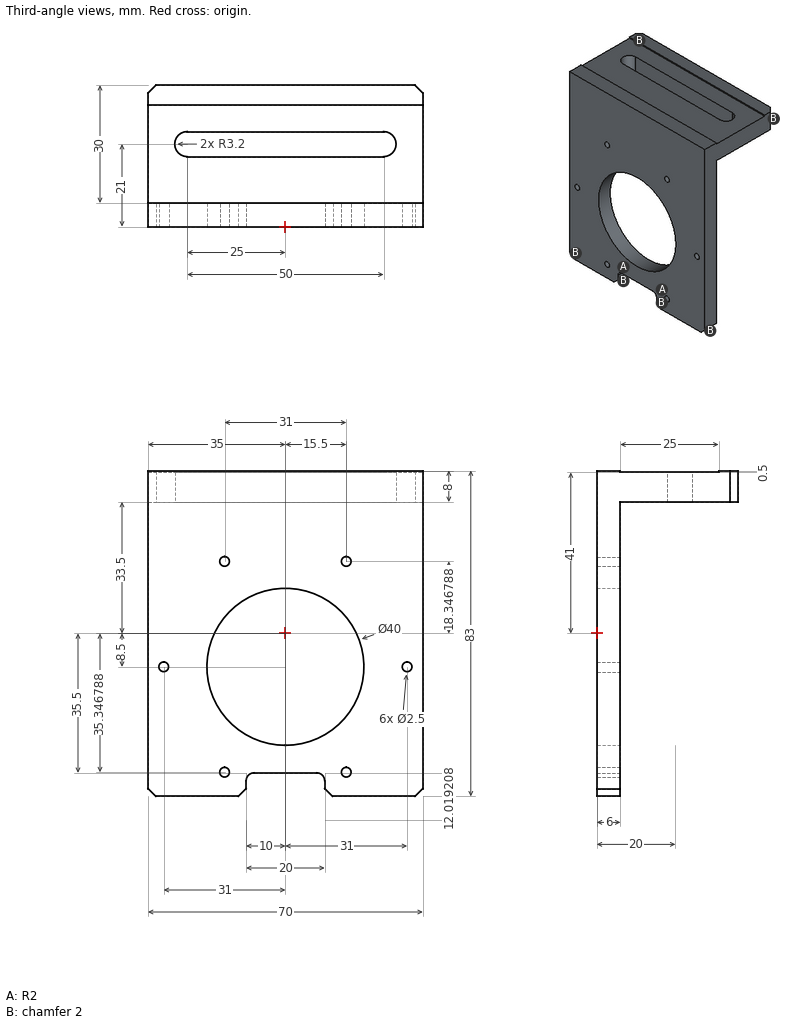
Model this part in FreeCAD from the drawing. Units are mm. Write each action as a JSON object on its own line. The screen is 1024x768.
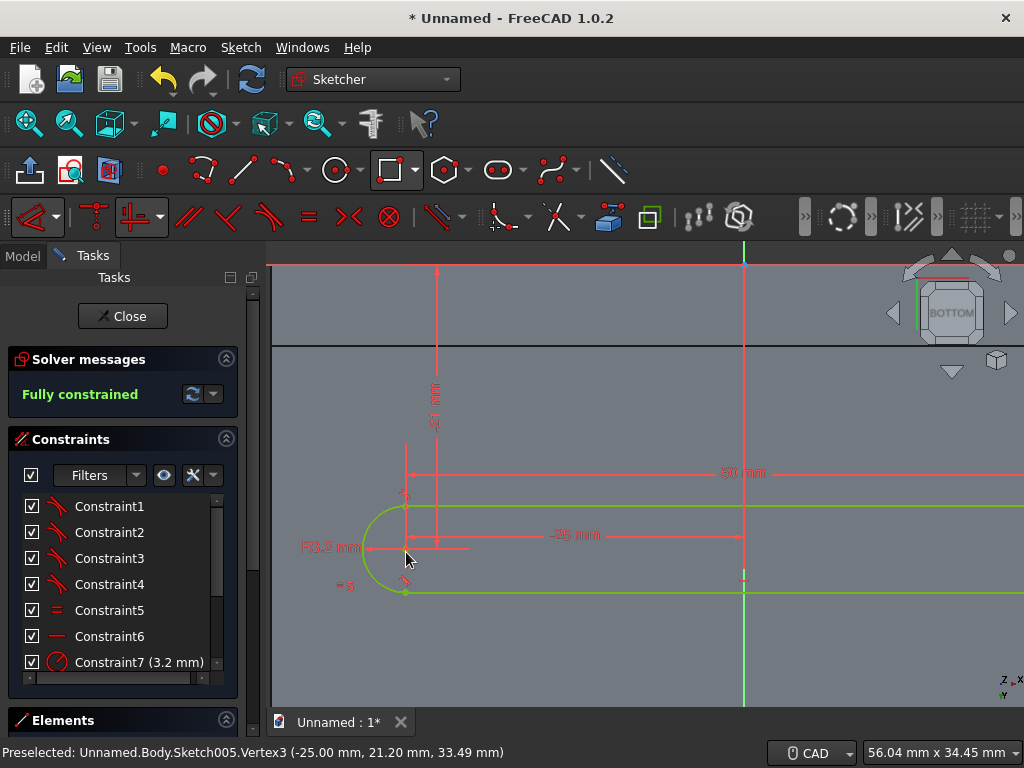
{"action": "left_click", "coordinate": [123, 316]}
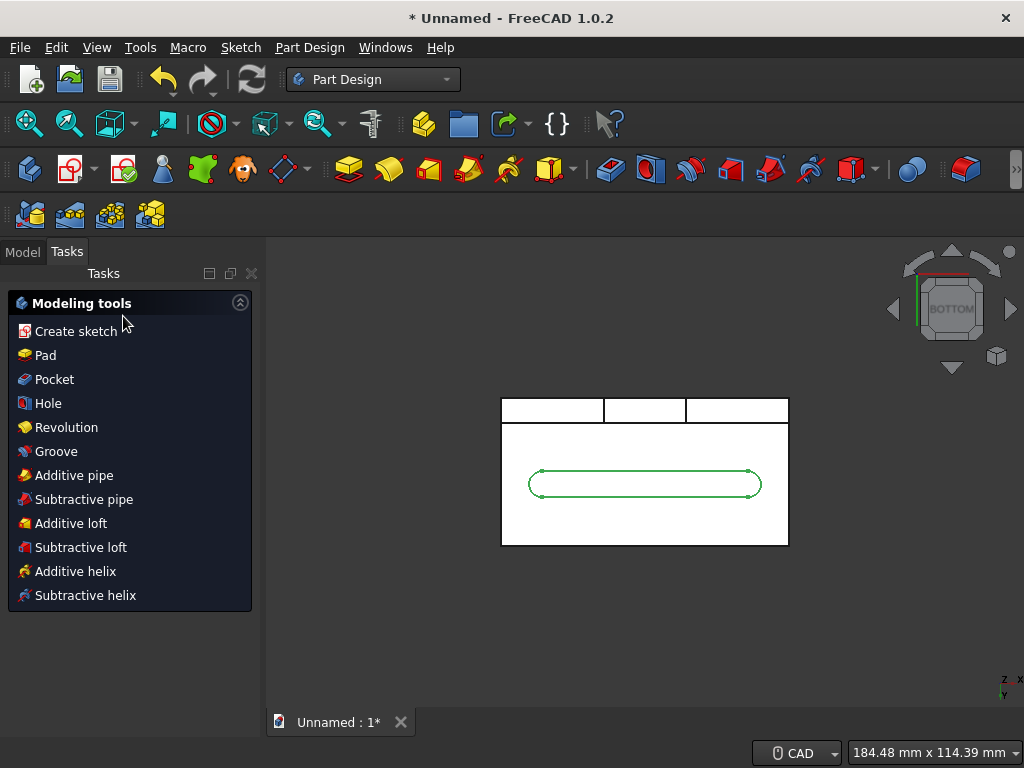
{"action": "left_click", "coordinate": [612, 170]}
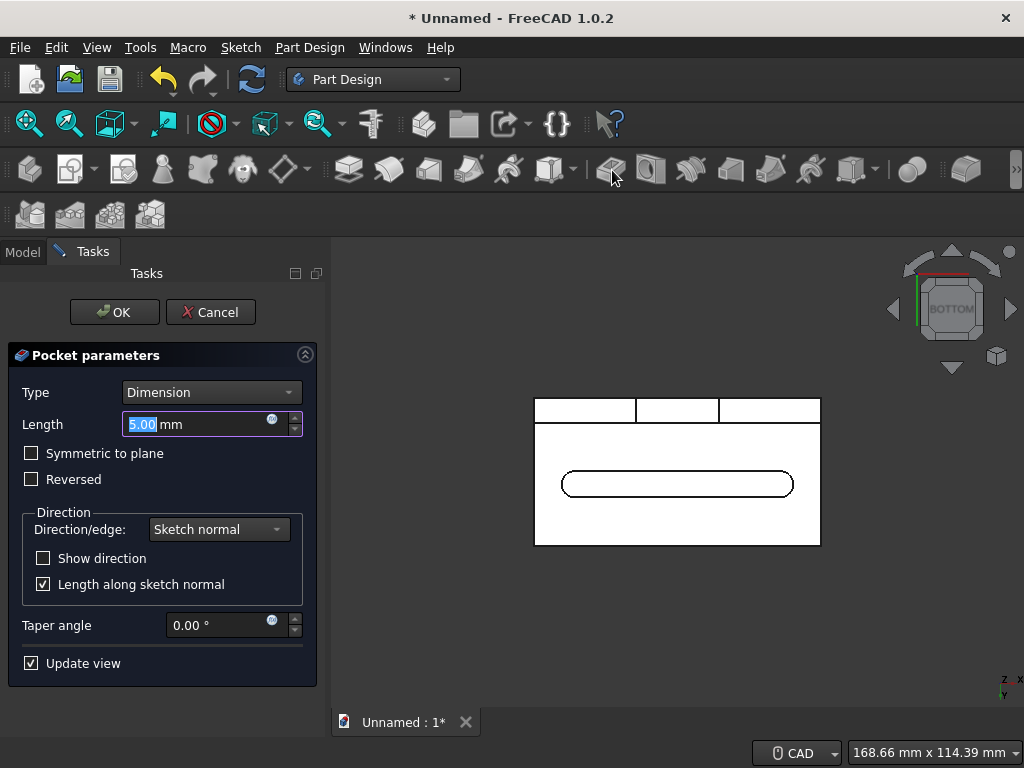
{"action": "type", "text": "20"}
{"action": "key", "text": "Tab"}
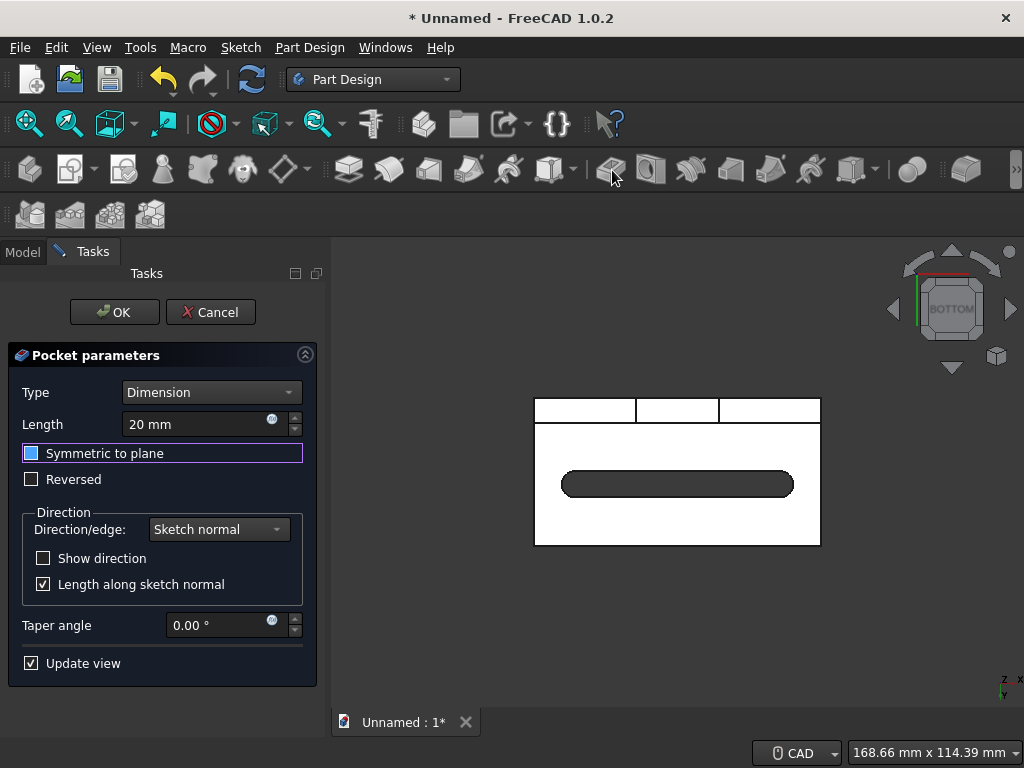
{"action": "left_click", "coordinate": [115, 312]}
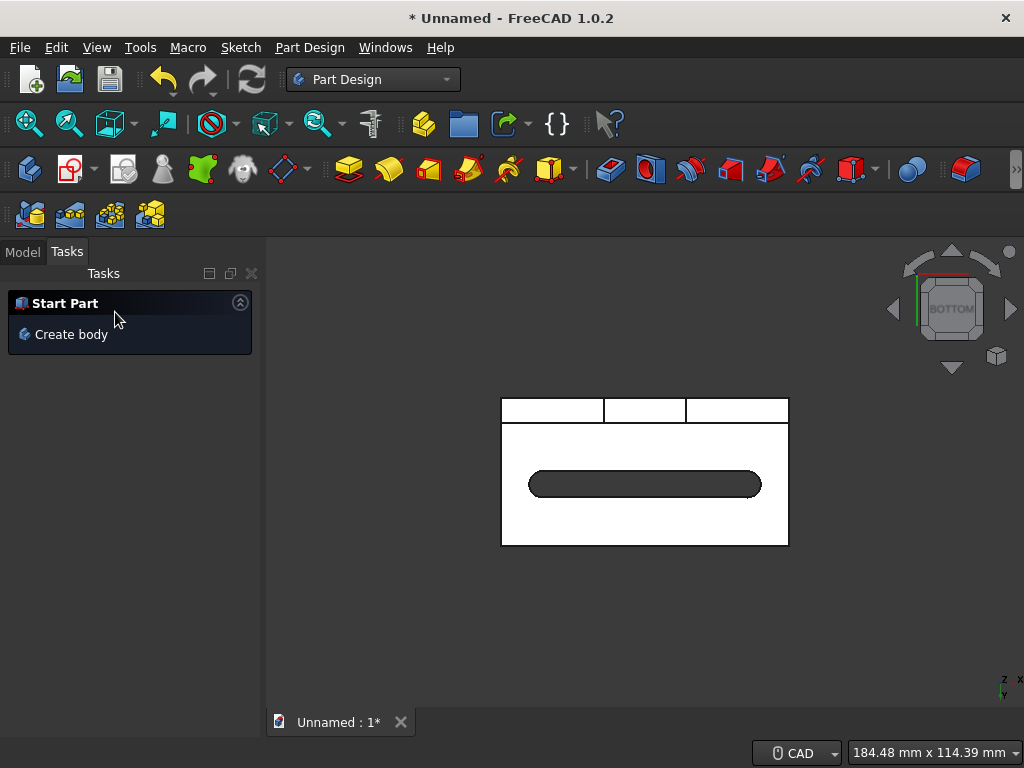
{"action": "left_click", "coordinate": [30, 124]}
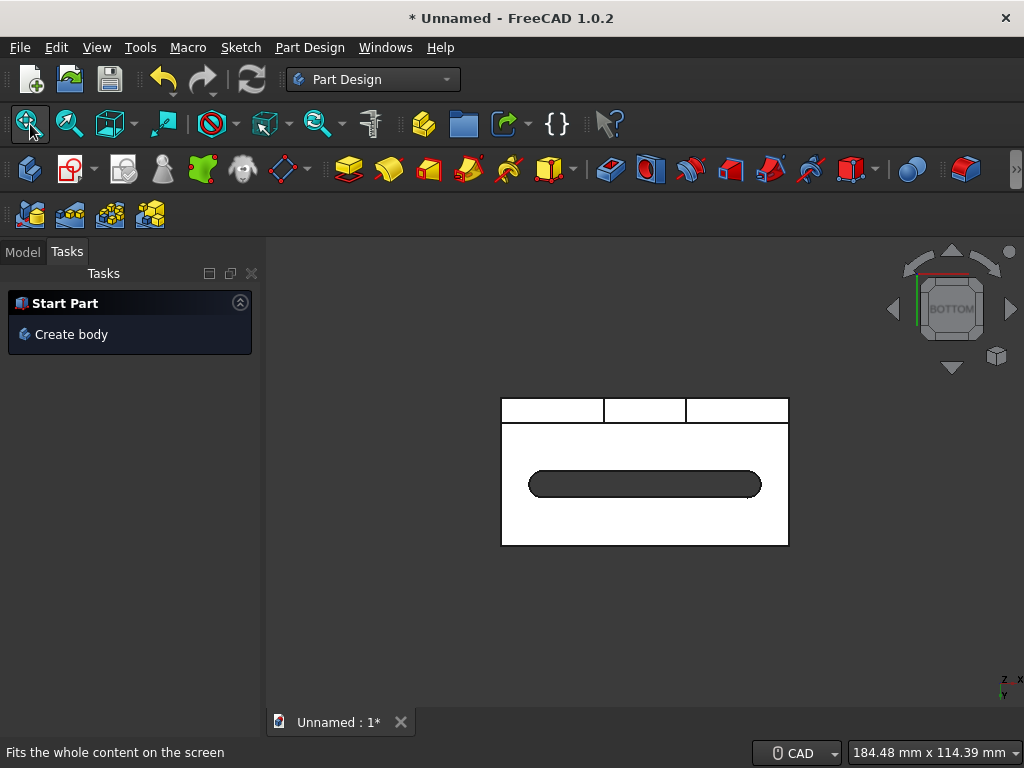
{"action": "key", "text": "6"}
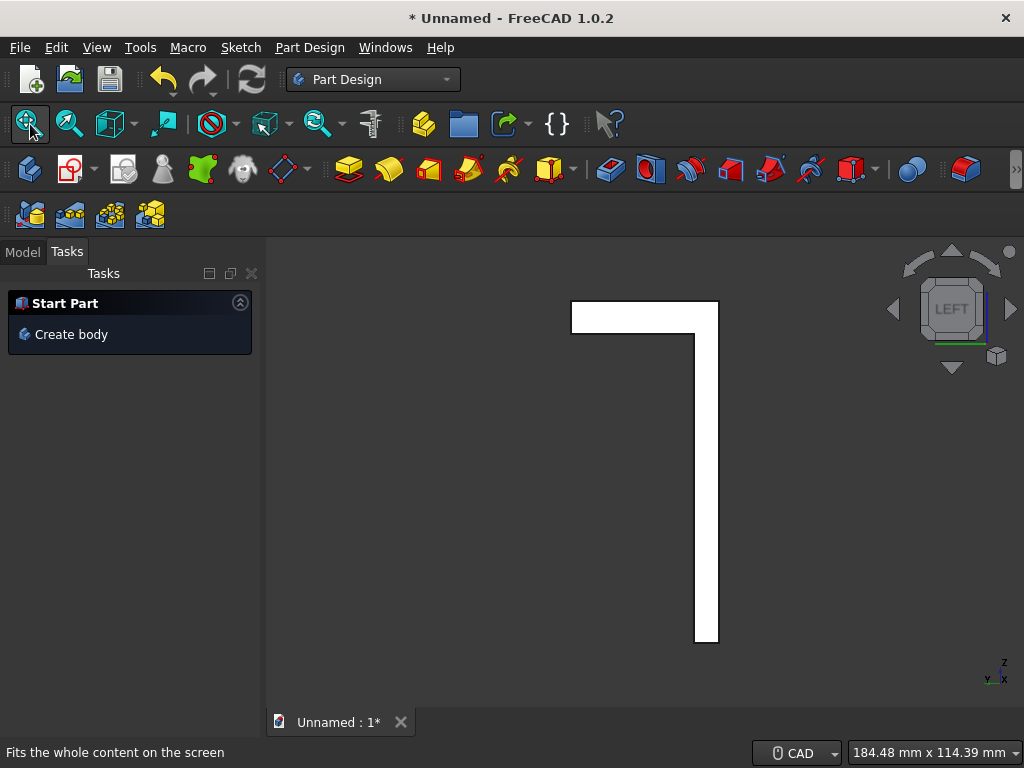
{"action": "left_click", "coordinate": [708, 617]}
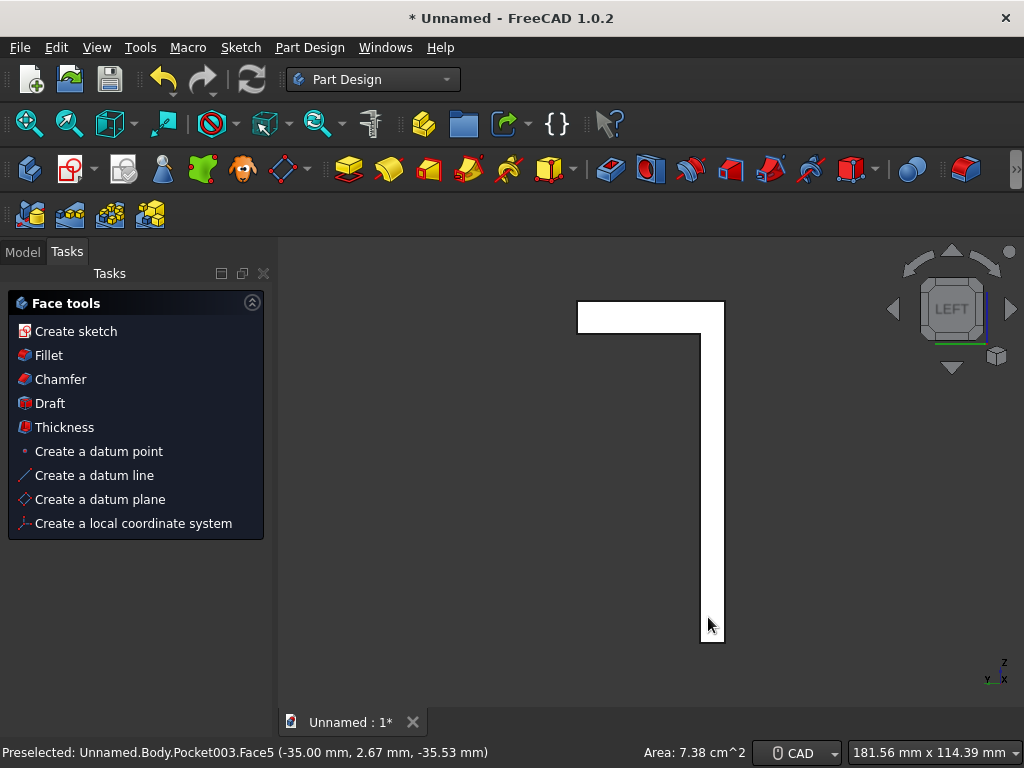
{"action": "left_click", "coordinate": [70, 170]}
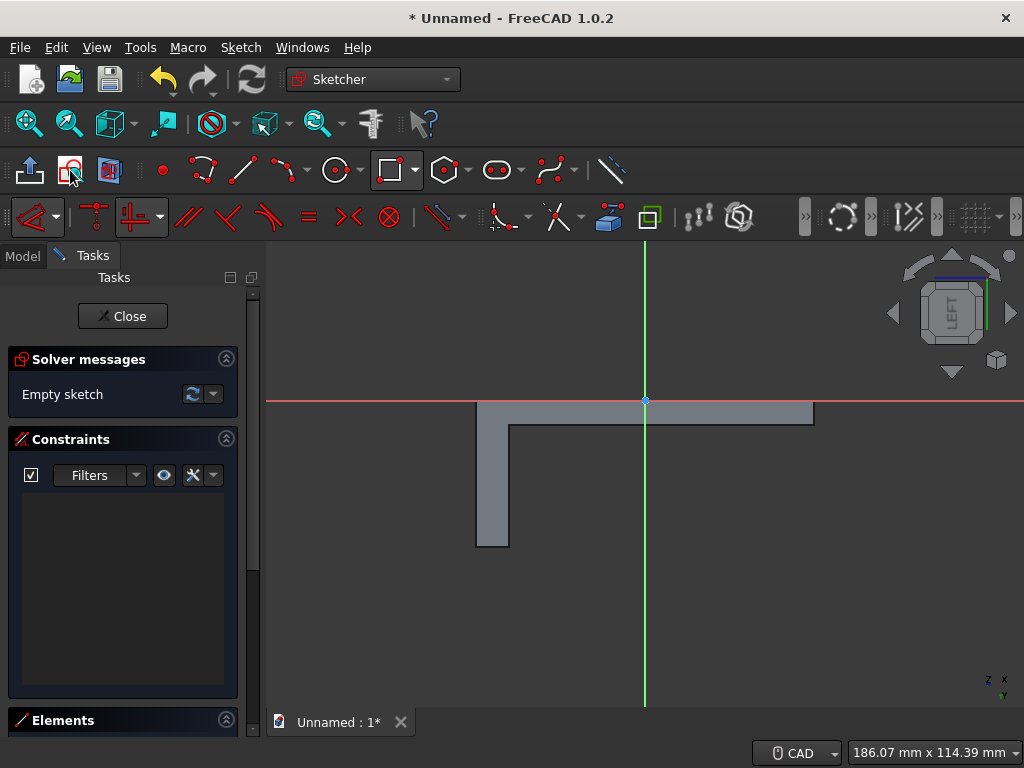
{"action": "scroll", "coordinate": [547, 456], "scroll_direction": "up", "scroll_amount": 4}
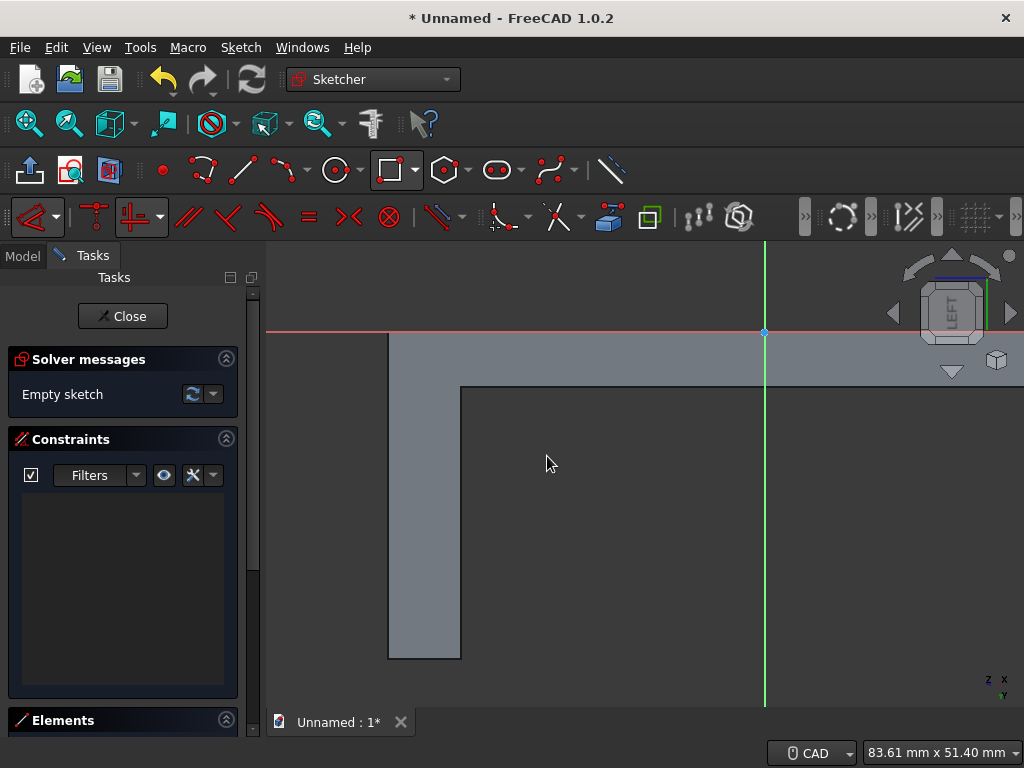
{"action": "left_click", "coordinate": [390, 170]}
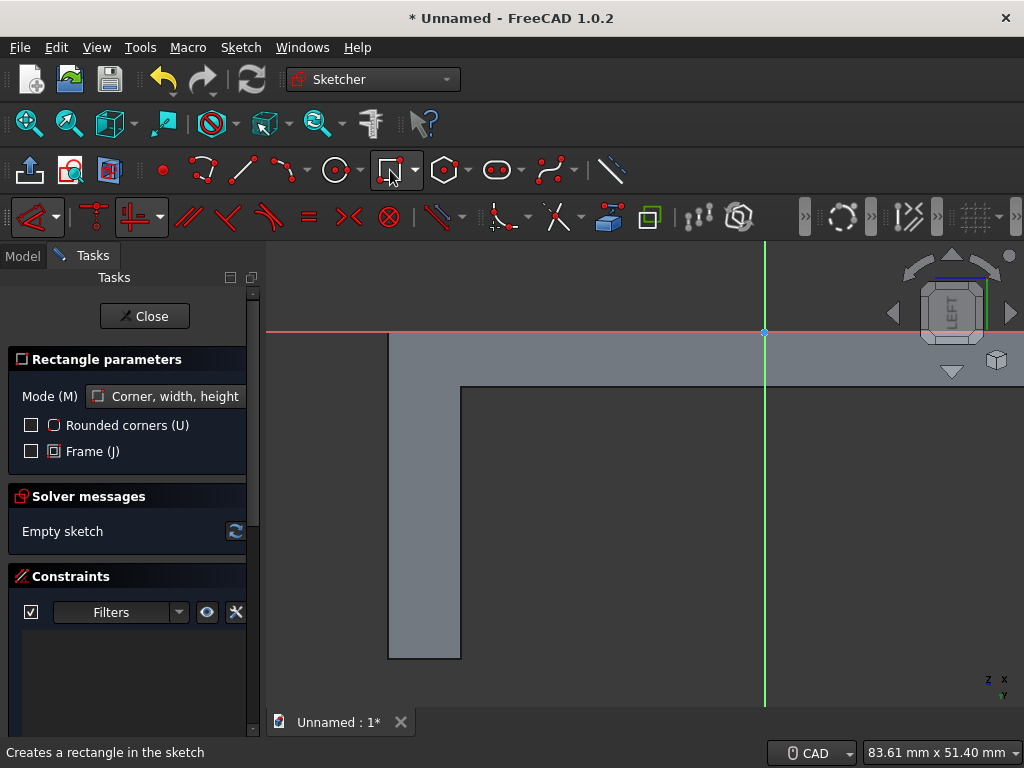
{"action": "scroll", "coordinate": [388, 387], "scroll_direction": "up", "scroll_amount": 7}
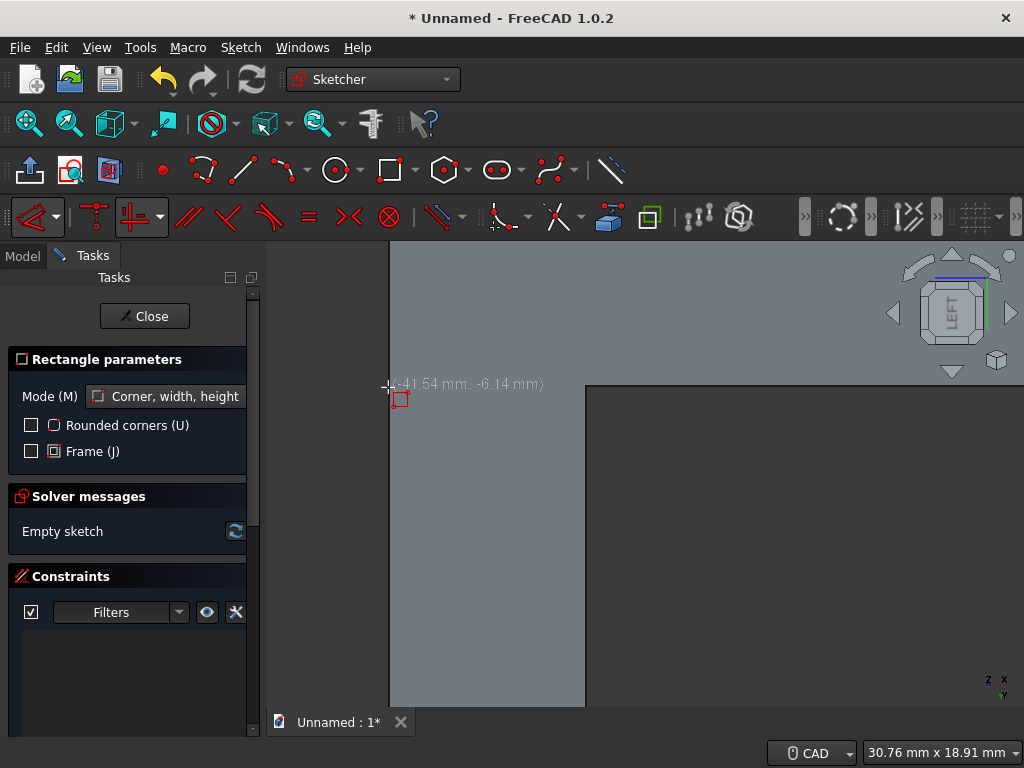
{"action": "scroll", "coordinate": [388, 389], "scroll_direction": "down", "scroll_amount": 7}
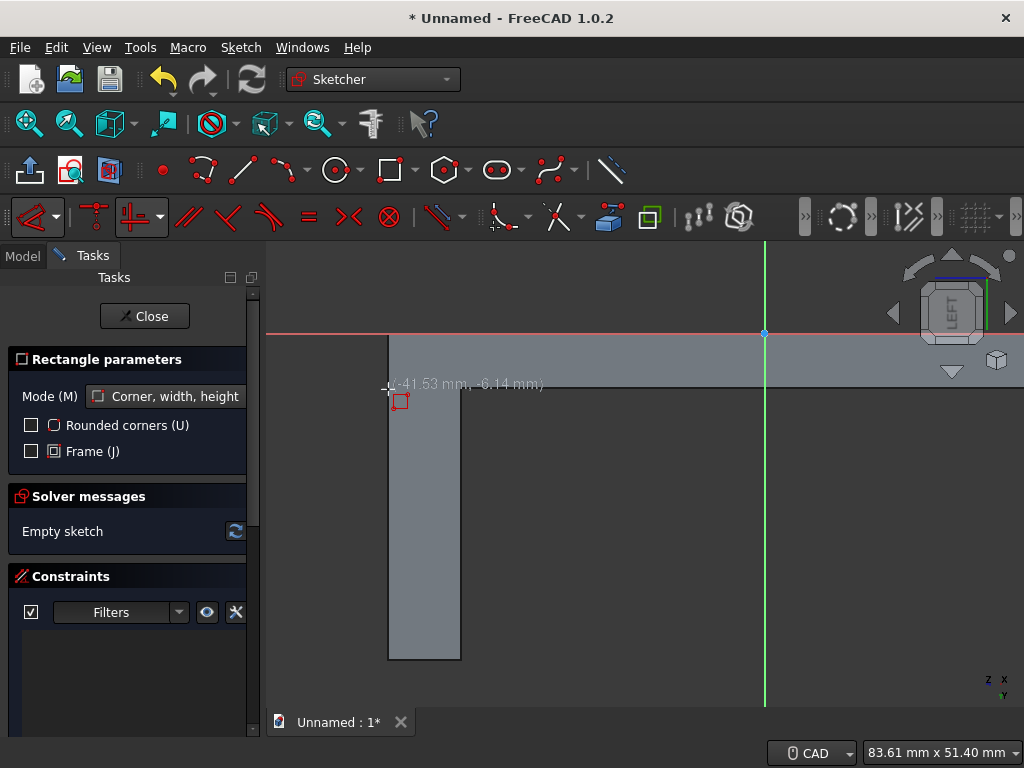
{"action": "left_click", "coordinate": [388, 388]}
{"action": "mouse_move", "coordinate": [393, 615]}